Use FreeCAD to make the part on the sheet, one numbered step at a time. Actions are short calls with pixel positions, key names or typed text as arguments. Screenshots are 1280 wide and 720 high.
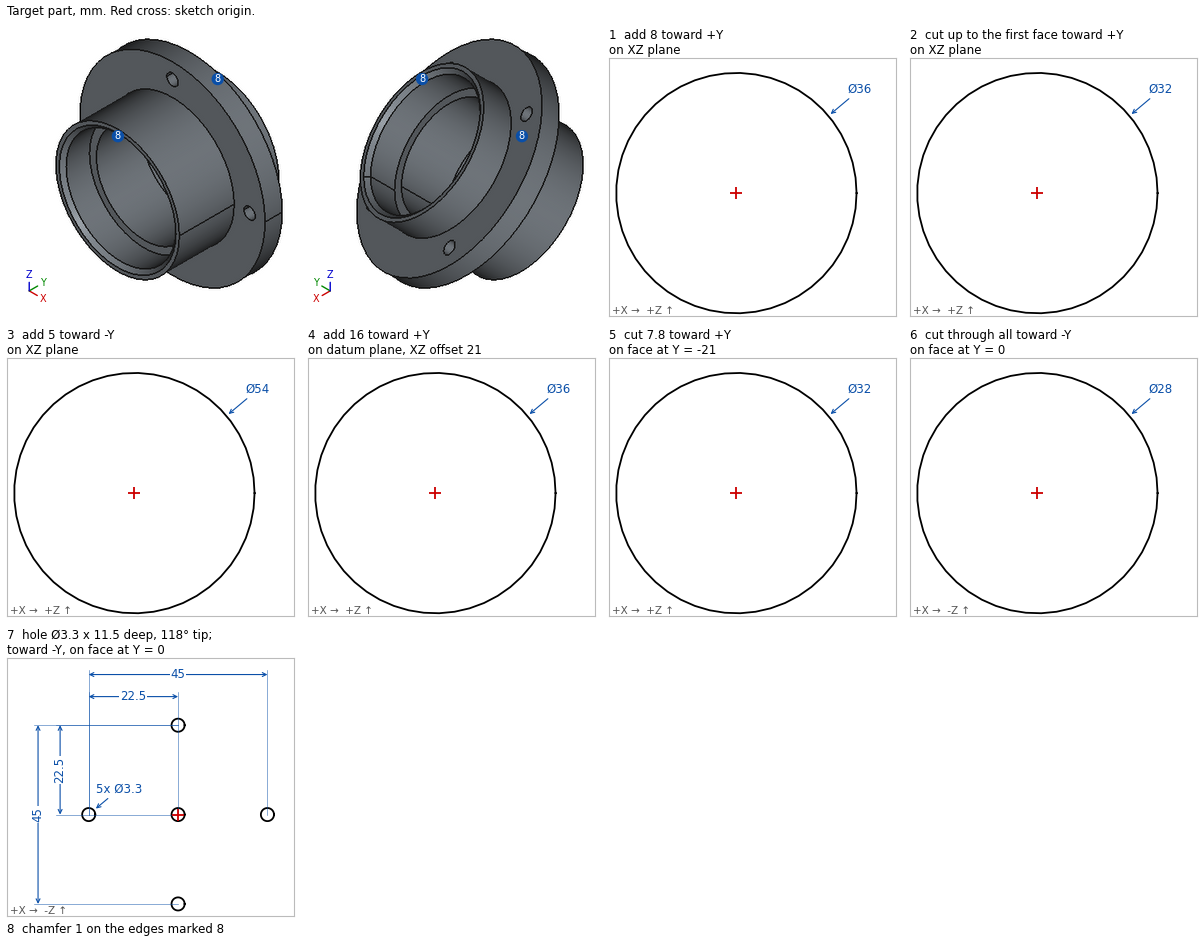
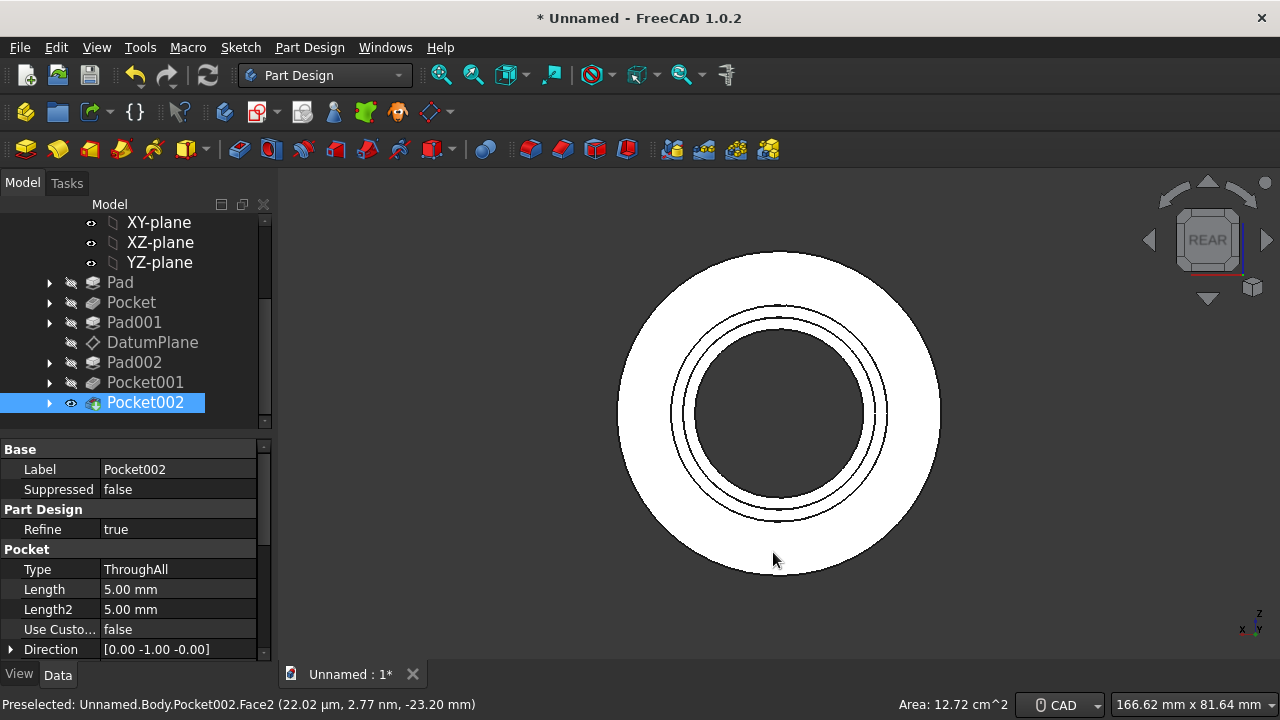
click(258, 112)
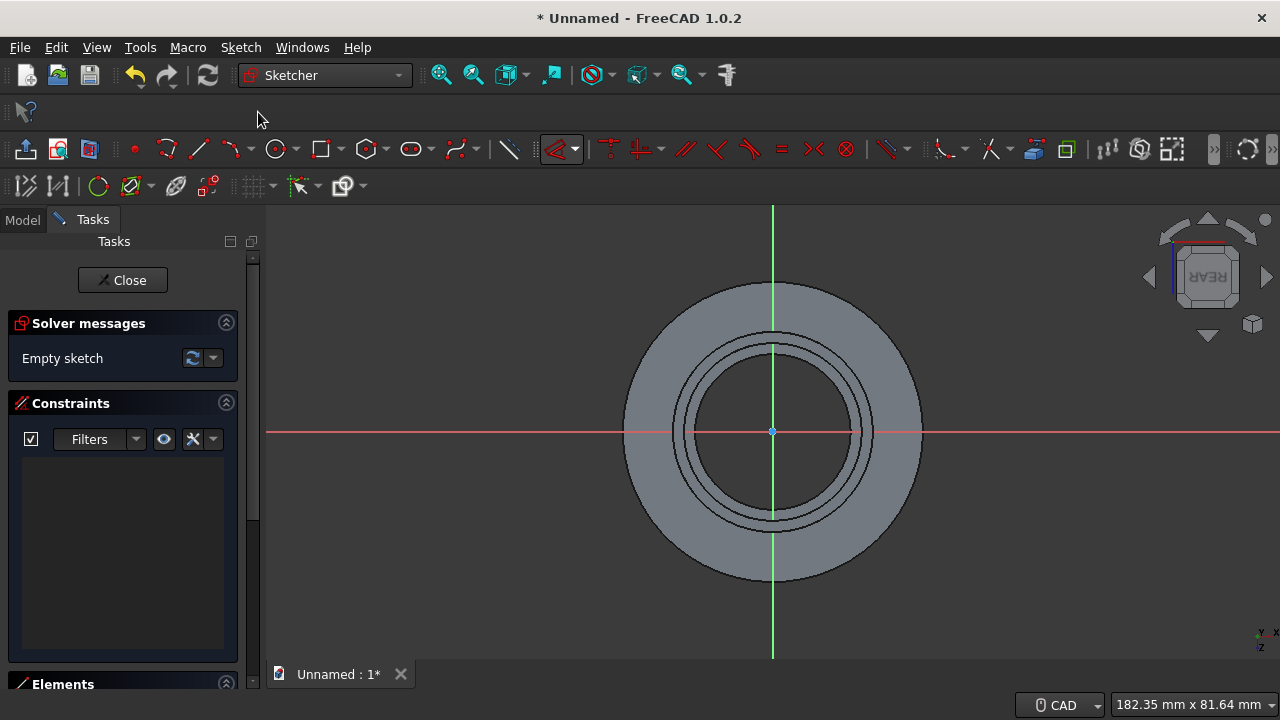
click(276, 150)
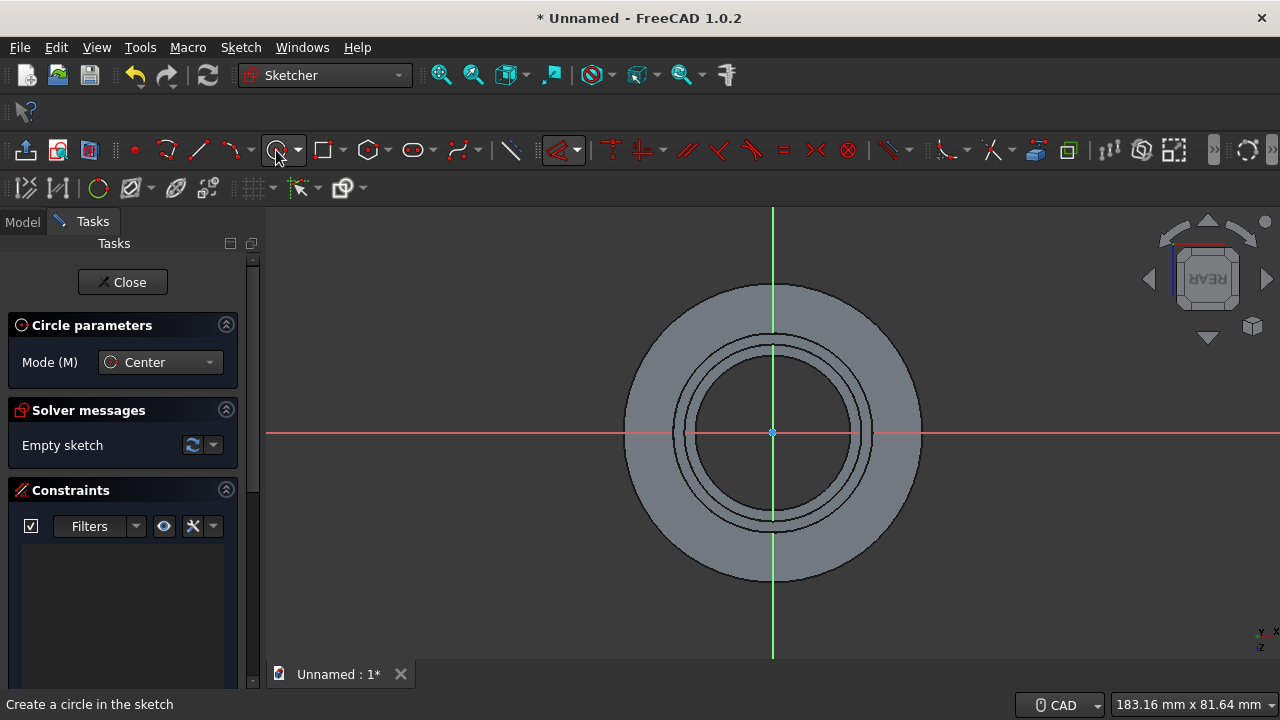
scroll(648, 433, up, 5)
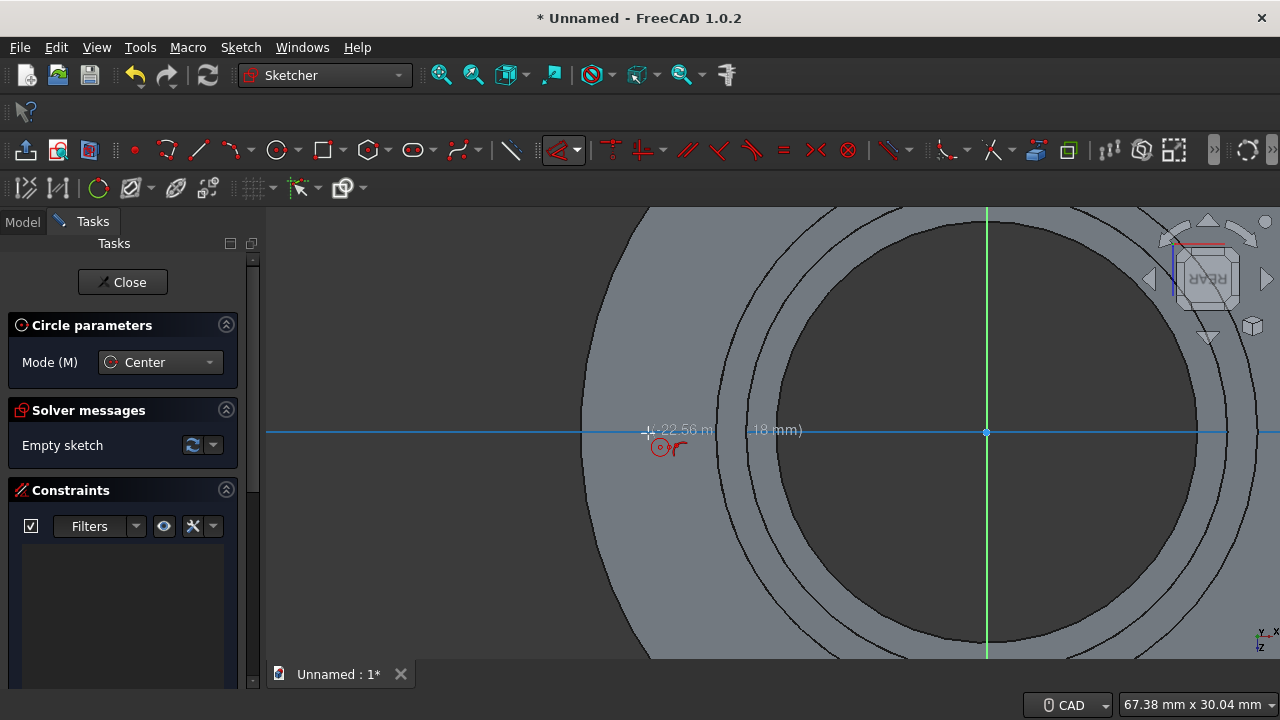
click(648, 432)
click(666, 415)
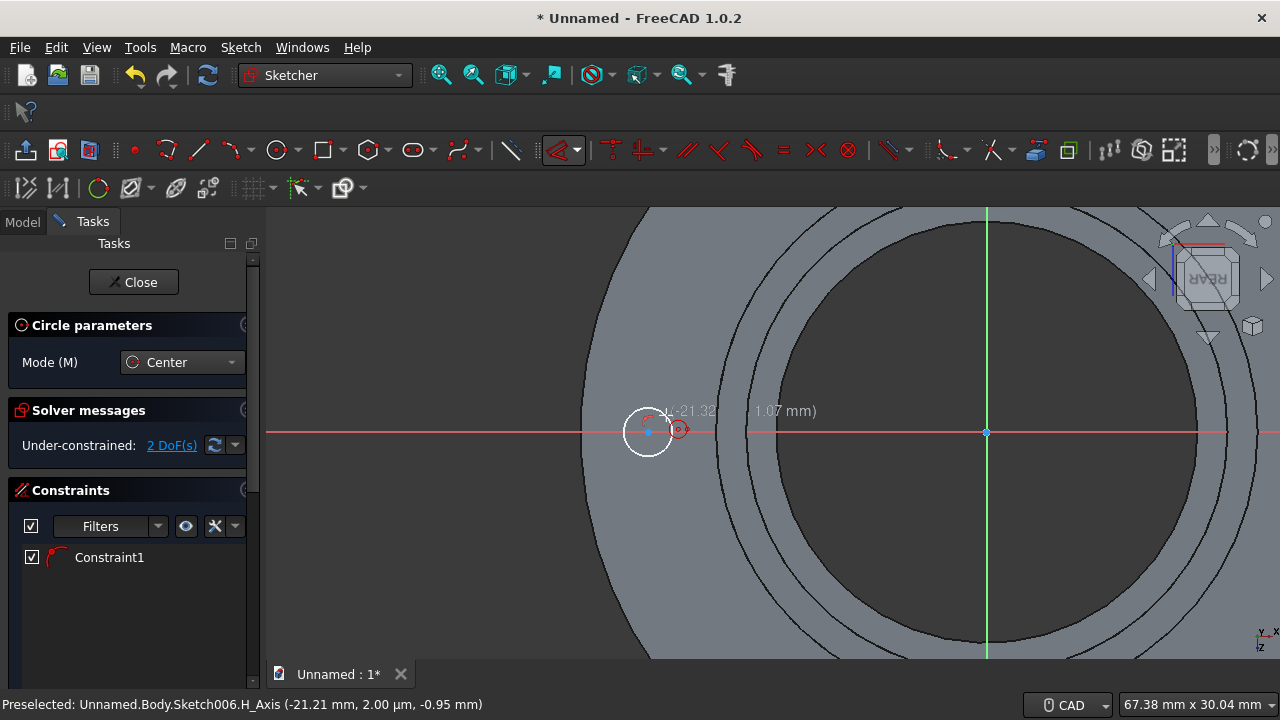
click(987, 432)
click(1004, 415)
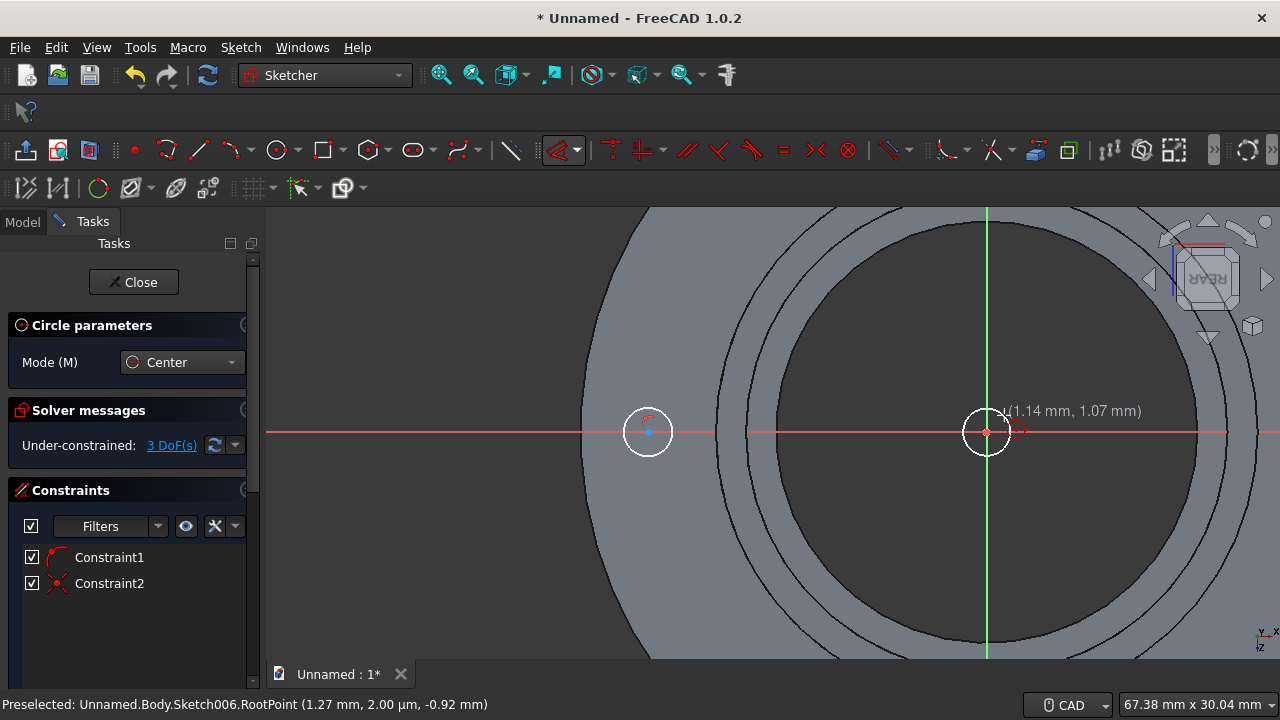
scroll(540, 434, down, 5)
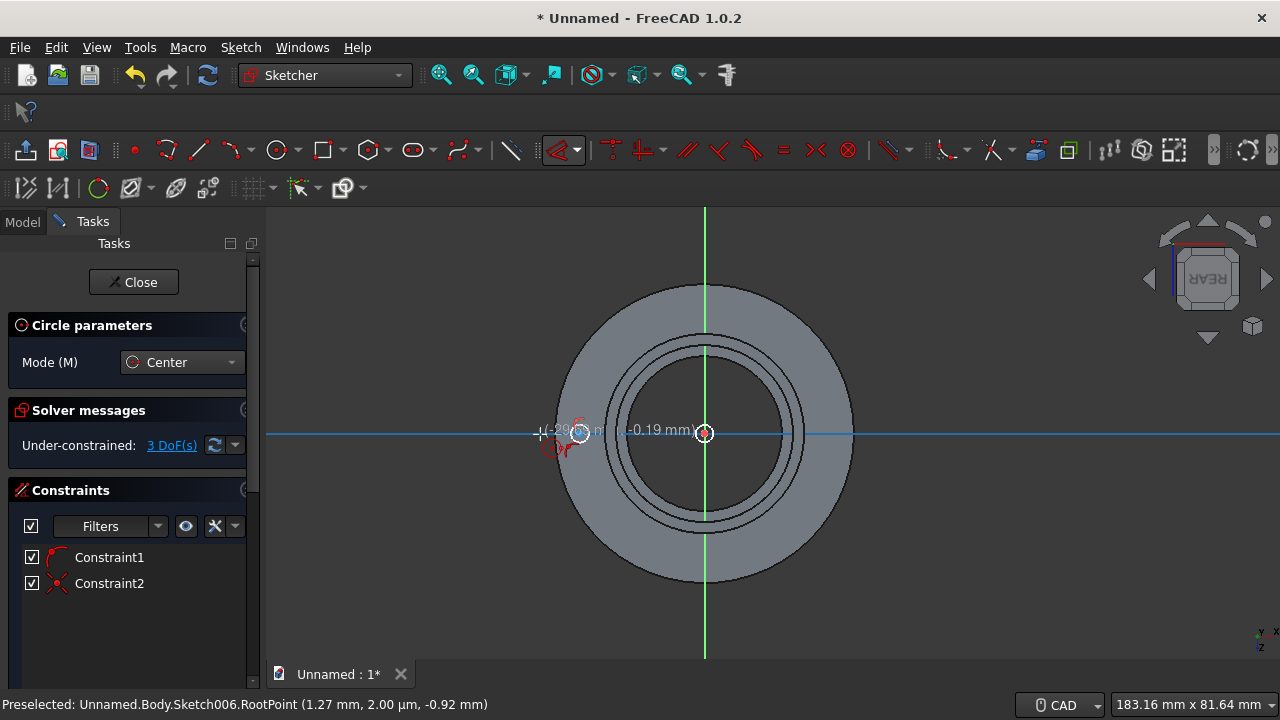
scroll(705, 309, up, 5)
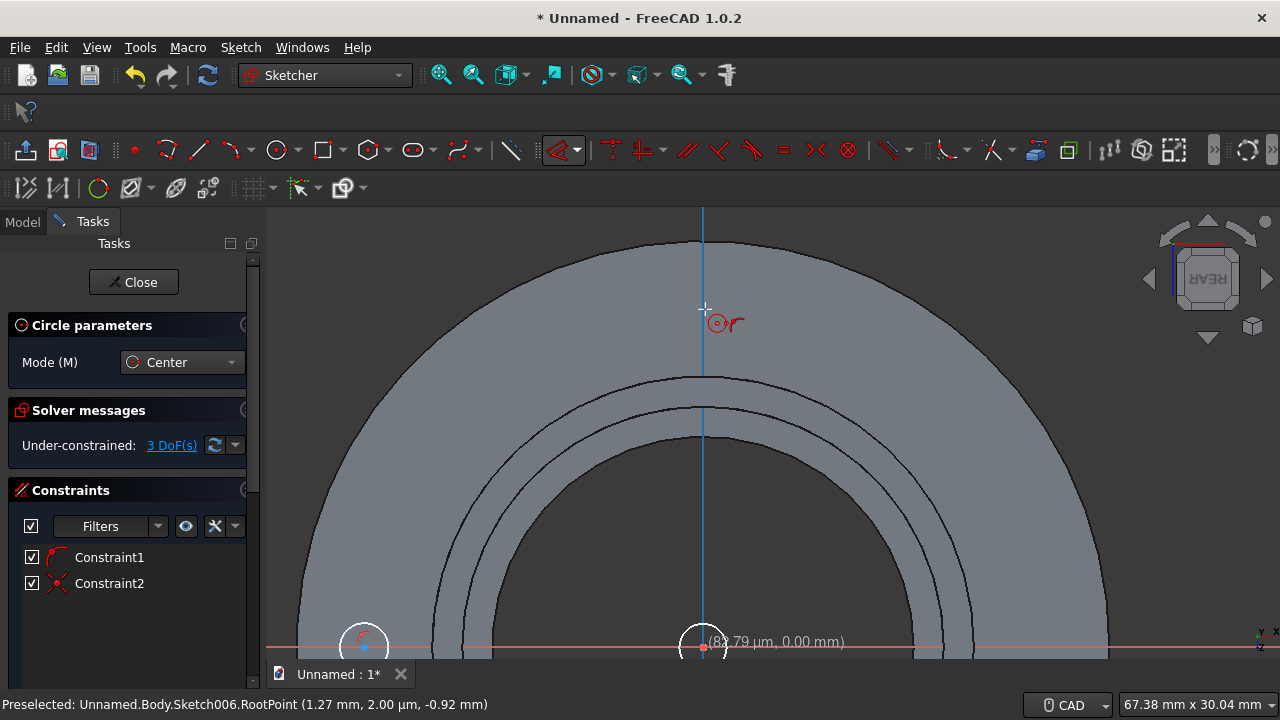
click(703, 309)
click(721, 291)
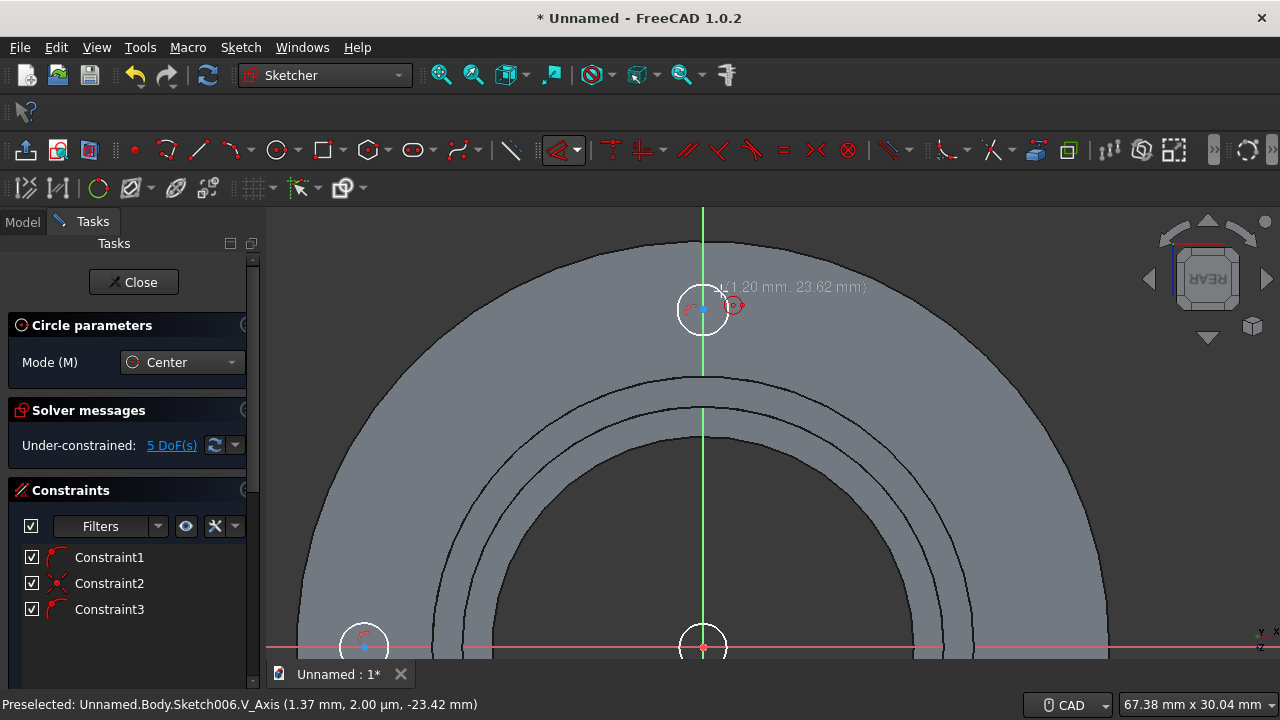
scroll(705, 308, down, 5)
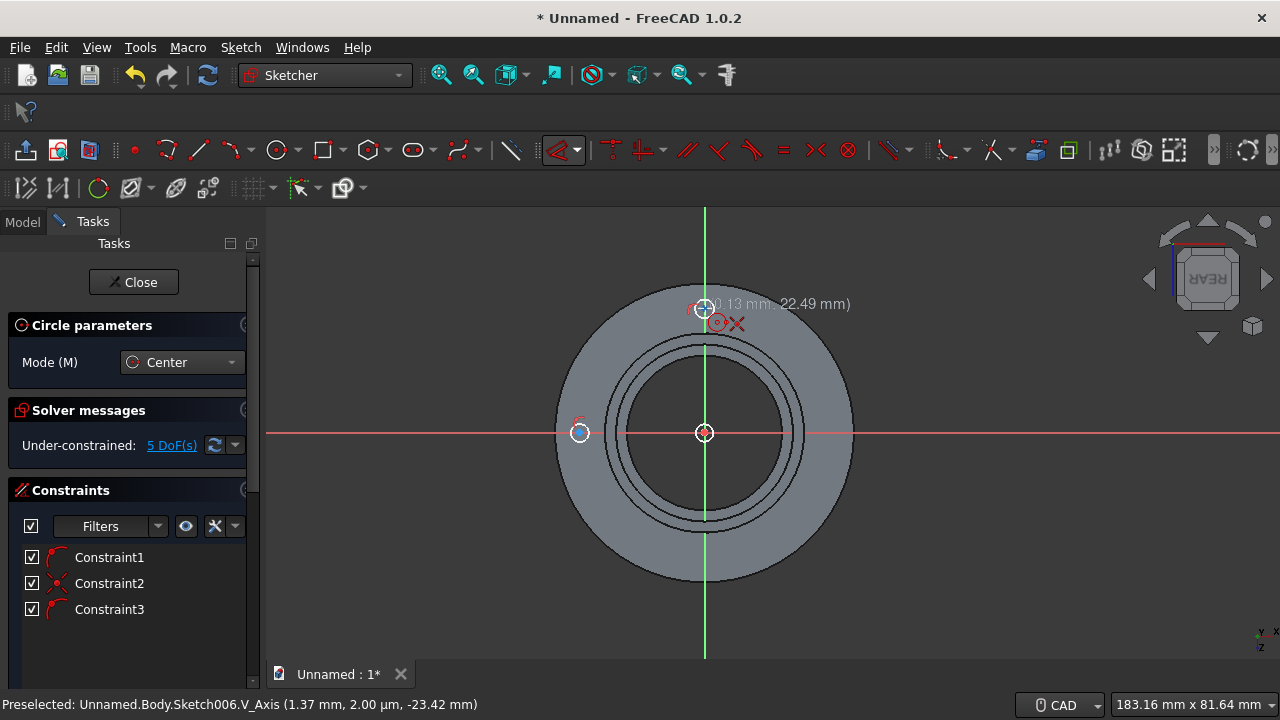
scroll(829, 433, up, 5)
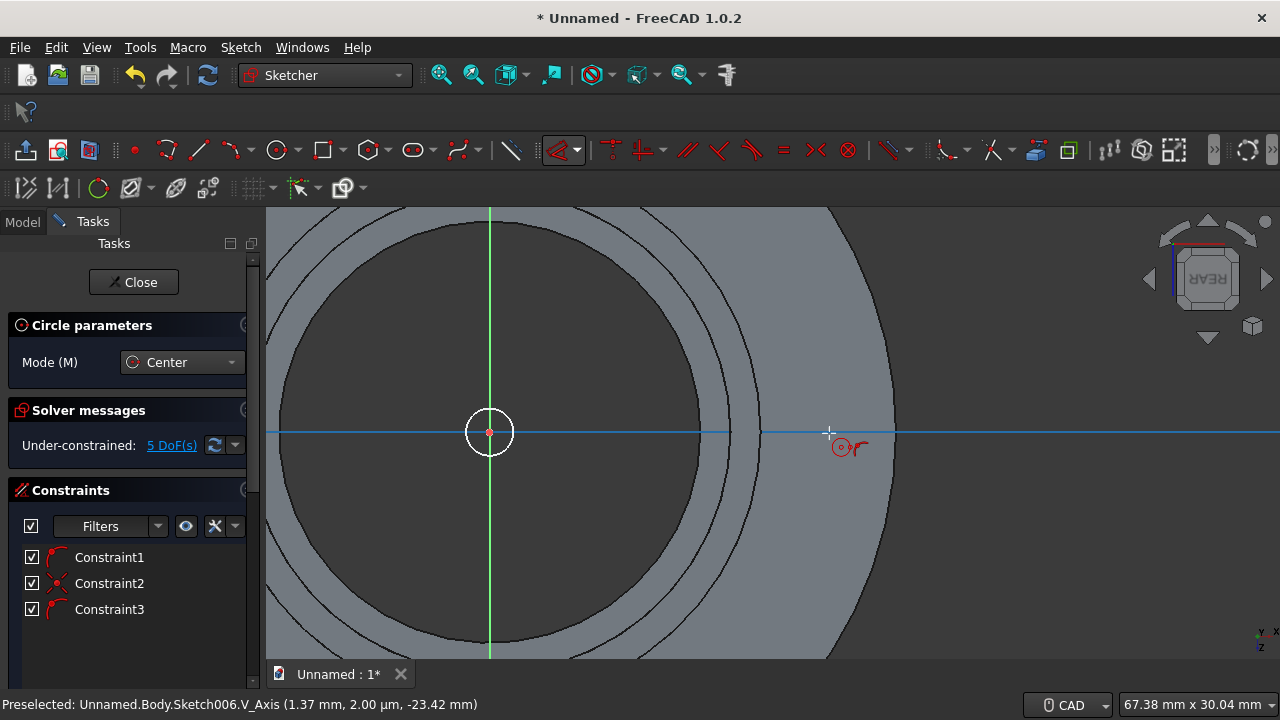
click(828, 432)
click(846, 415)